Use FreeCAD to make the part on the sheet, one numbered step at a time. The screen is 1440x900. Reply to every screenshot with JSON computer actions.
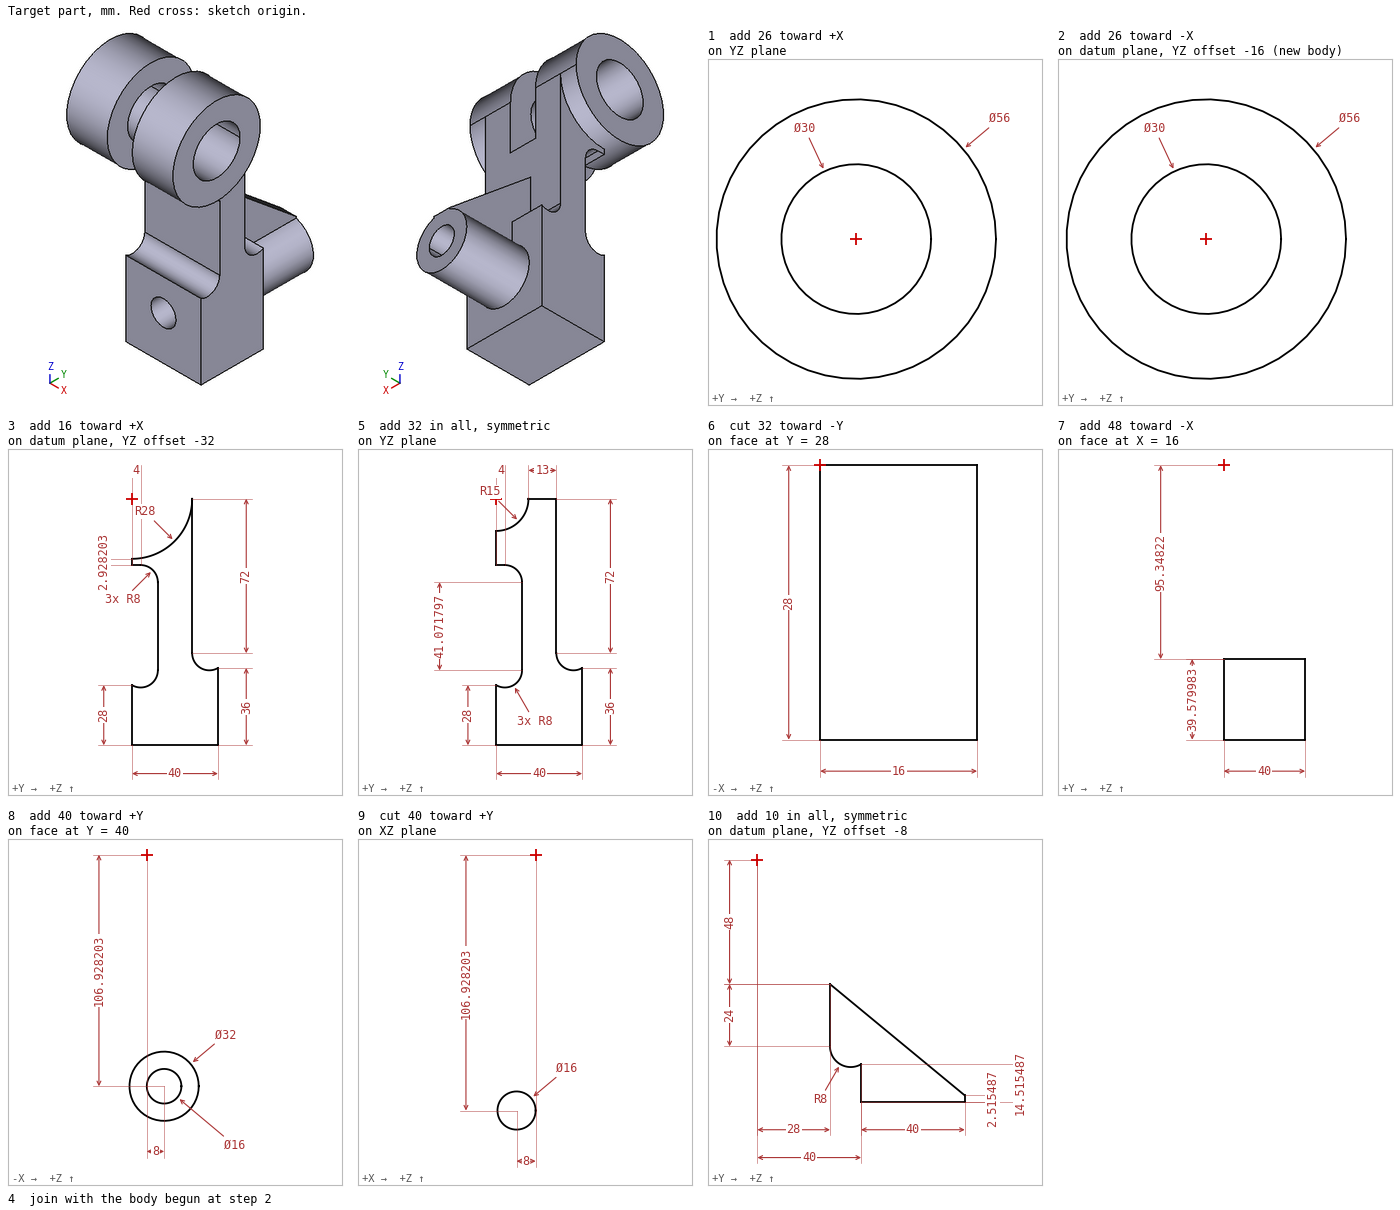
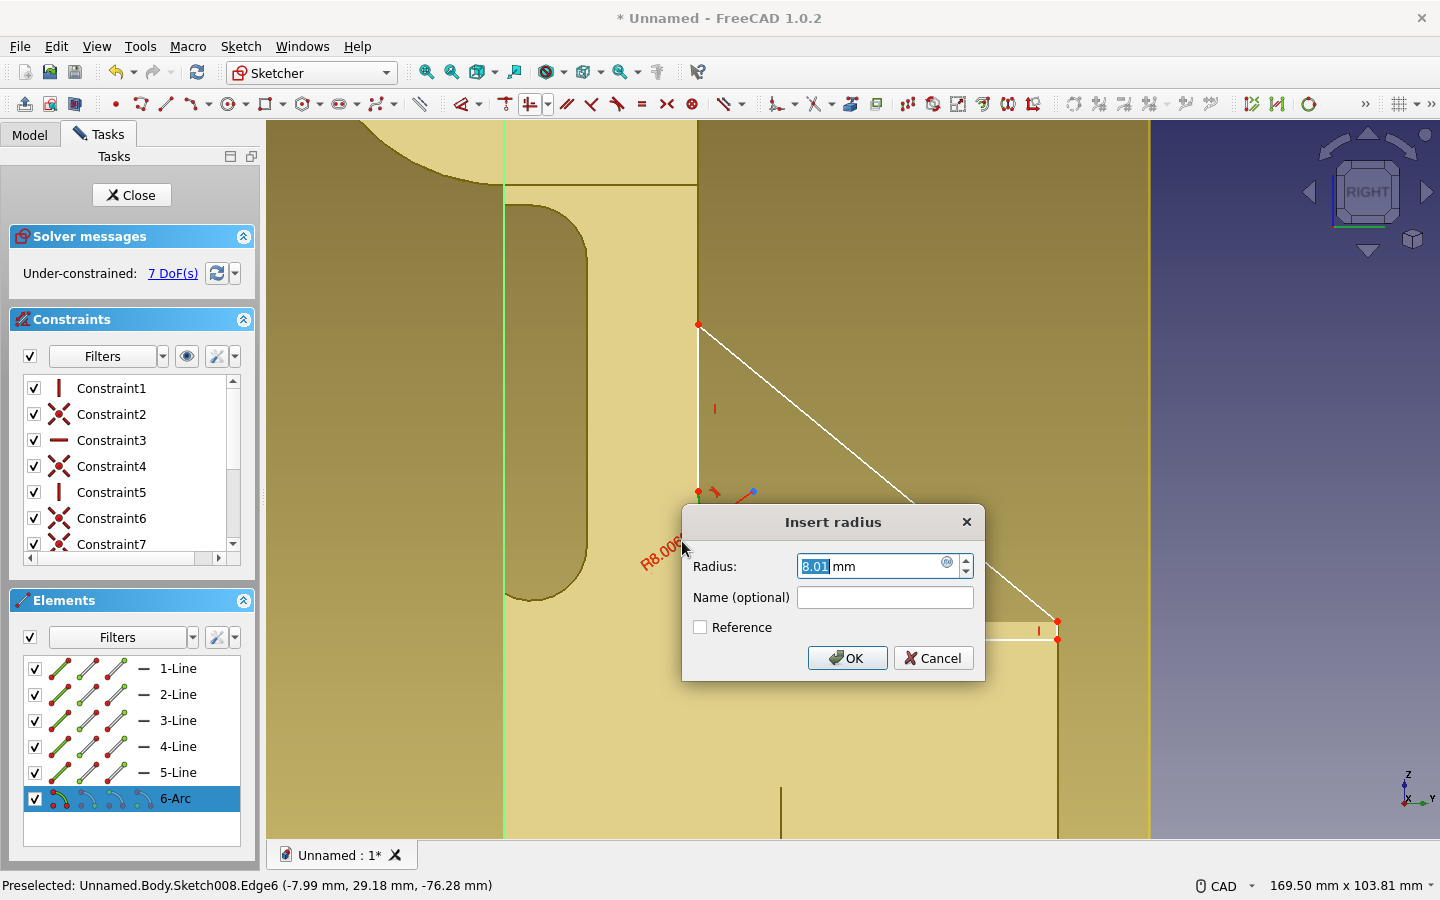
{"action": "type", "text": "8"}
{"action": "key", "text": "Return"}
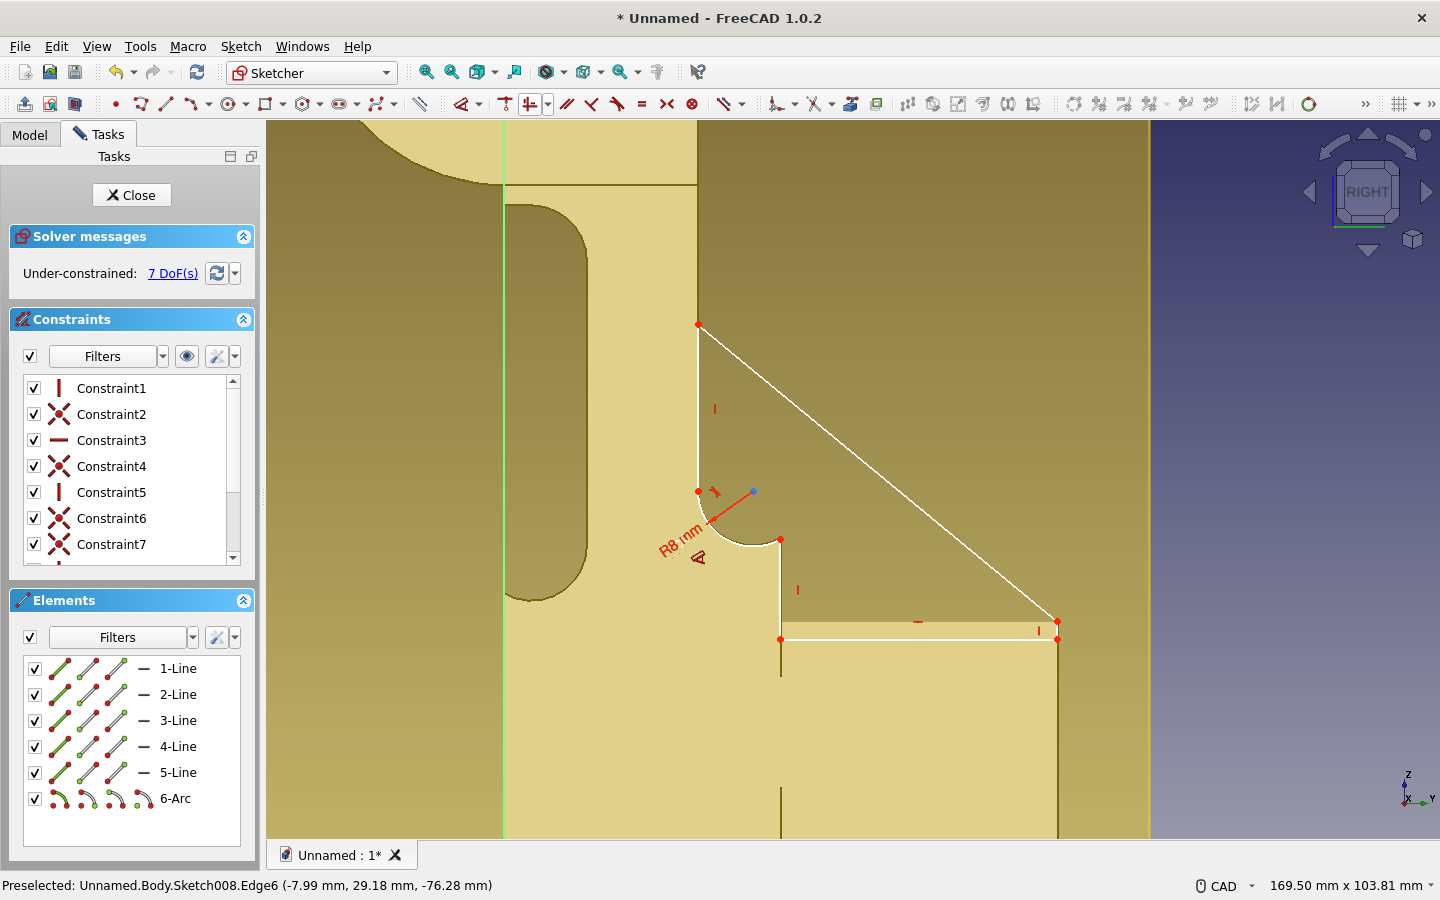
{"action": "left_click", "coordinate": [864, 640]}
{"action": "left_click", "coordinate": [919, 674]}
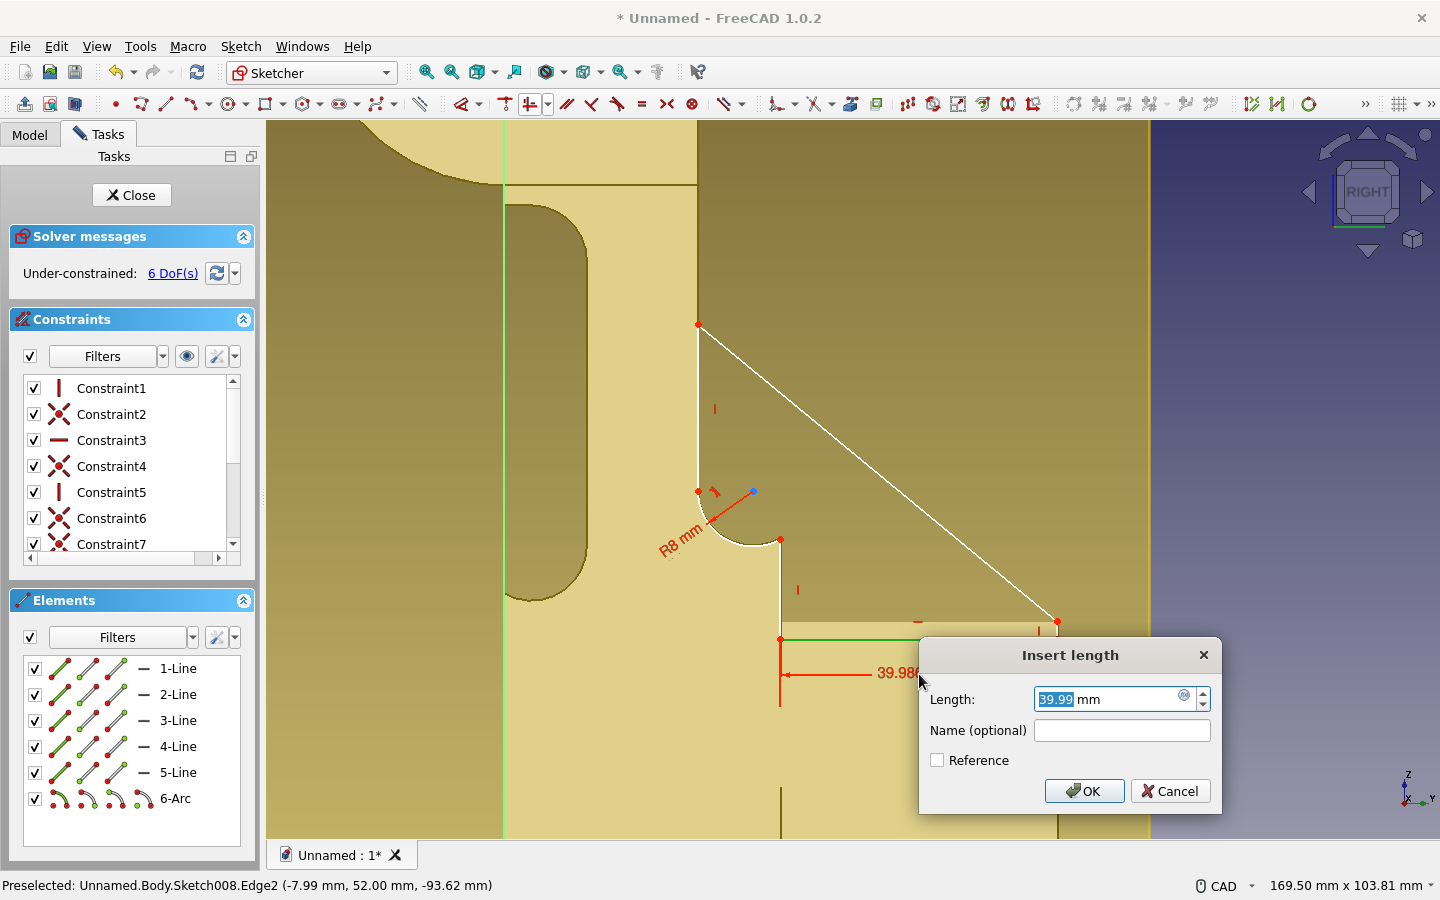
{"action": "type", "text": "40"}
{"action": "key", "text": "Return"}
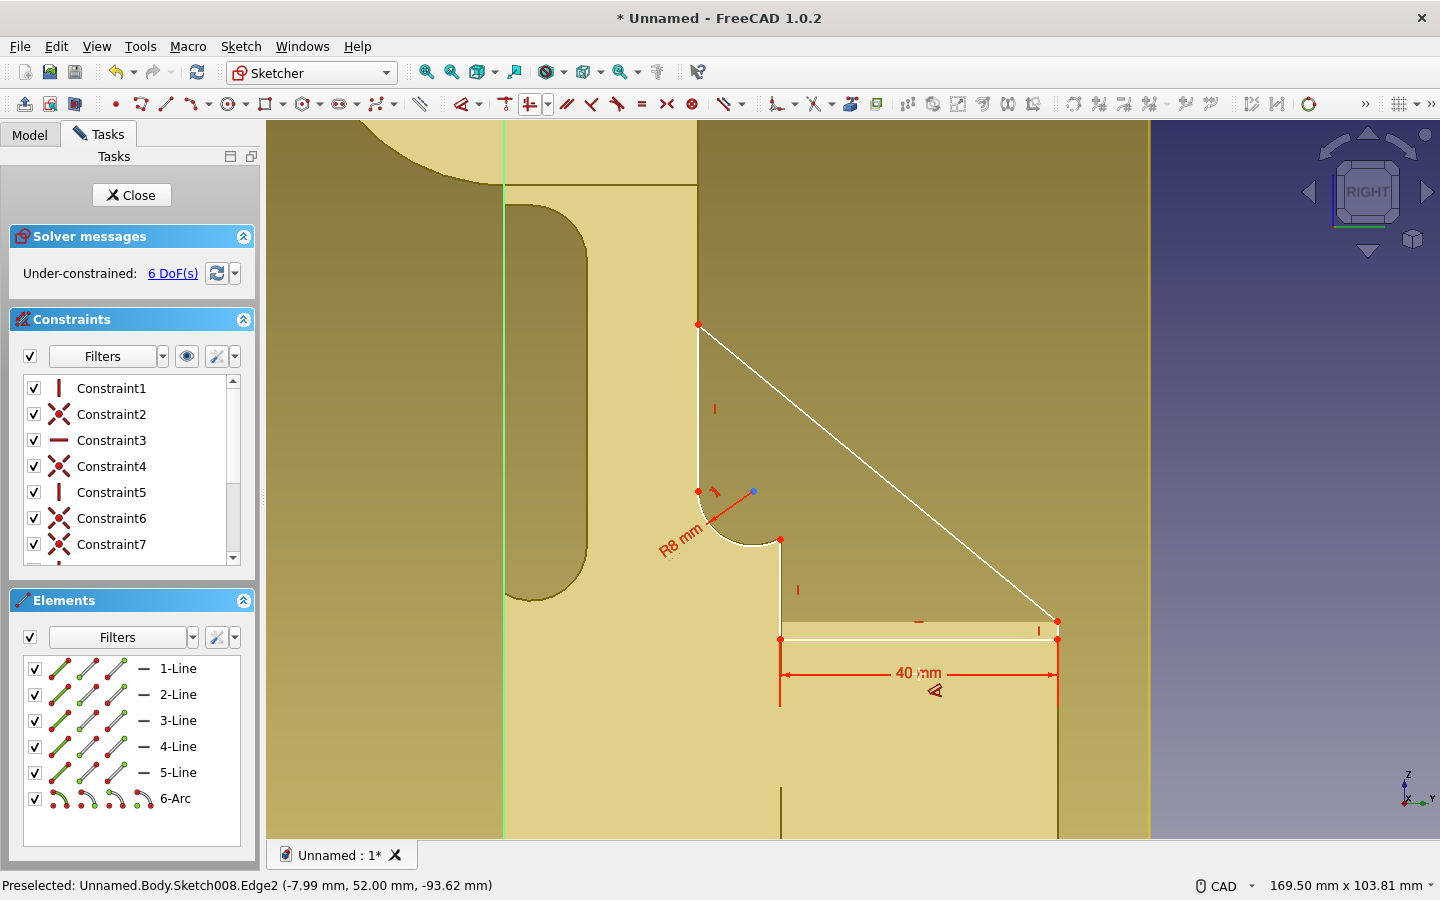
{"action": "left_click", "coordinate": [698, 375]}
{"action": "left_click", "coordinate": [664, 408]}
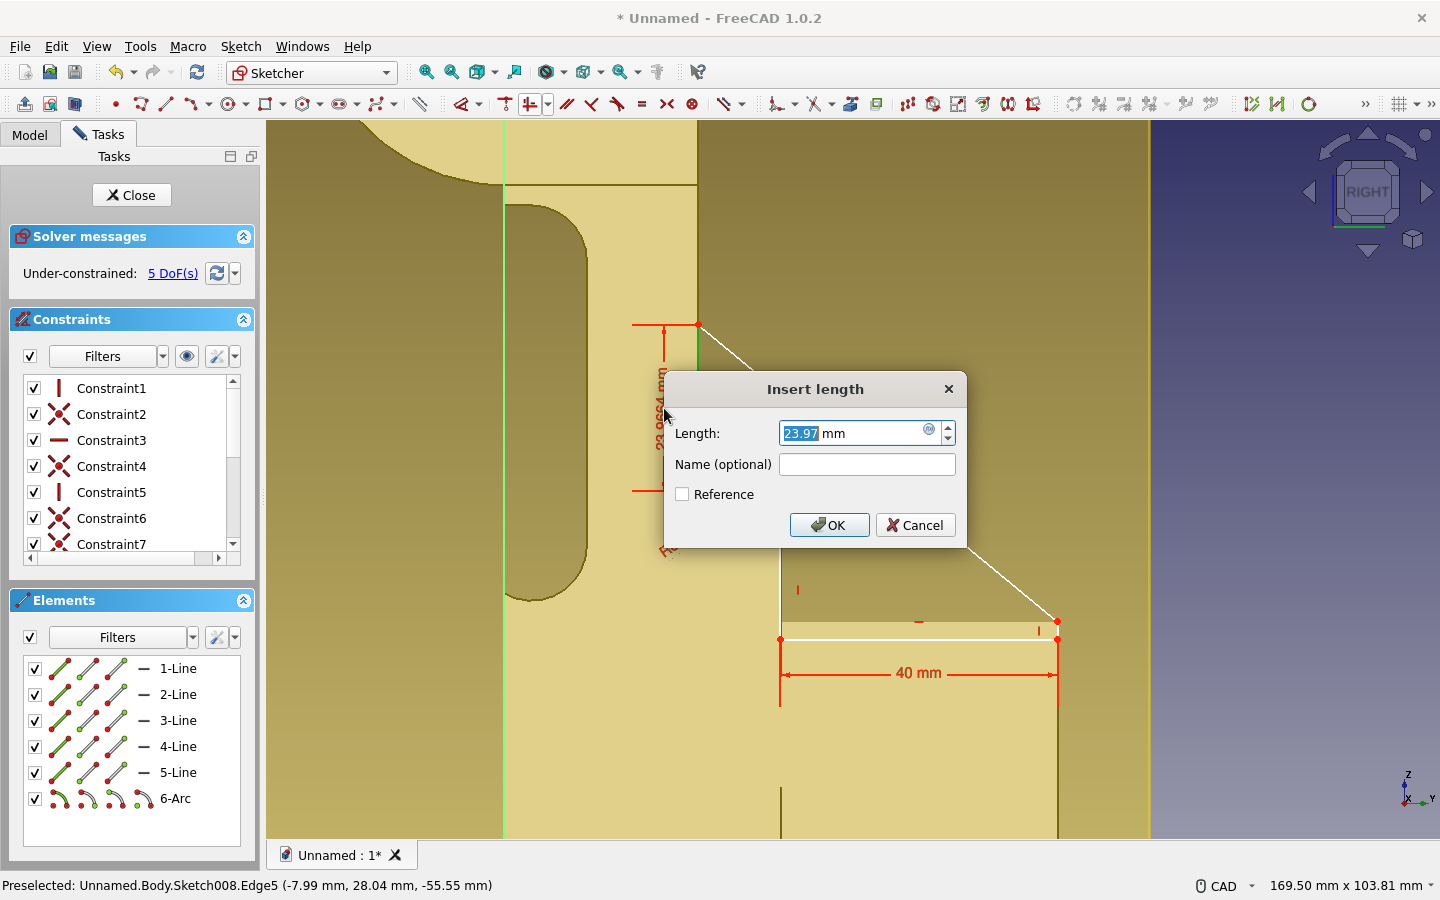
{"action": "type", "text": "24"}
{"action": "key", "text": "Return"}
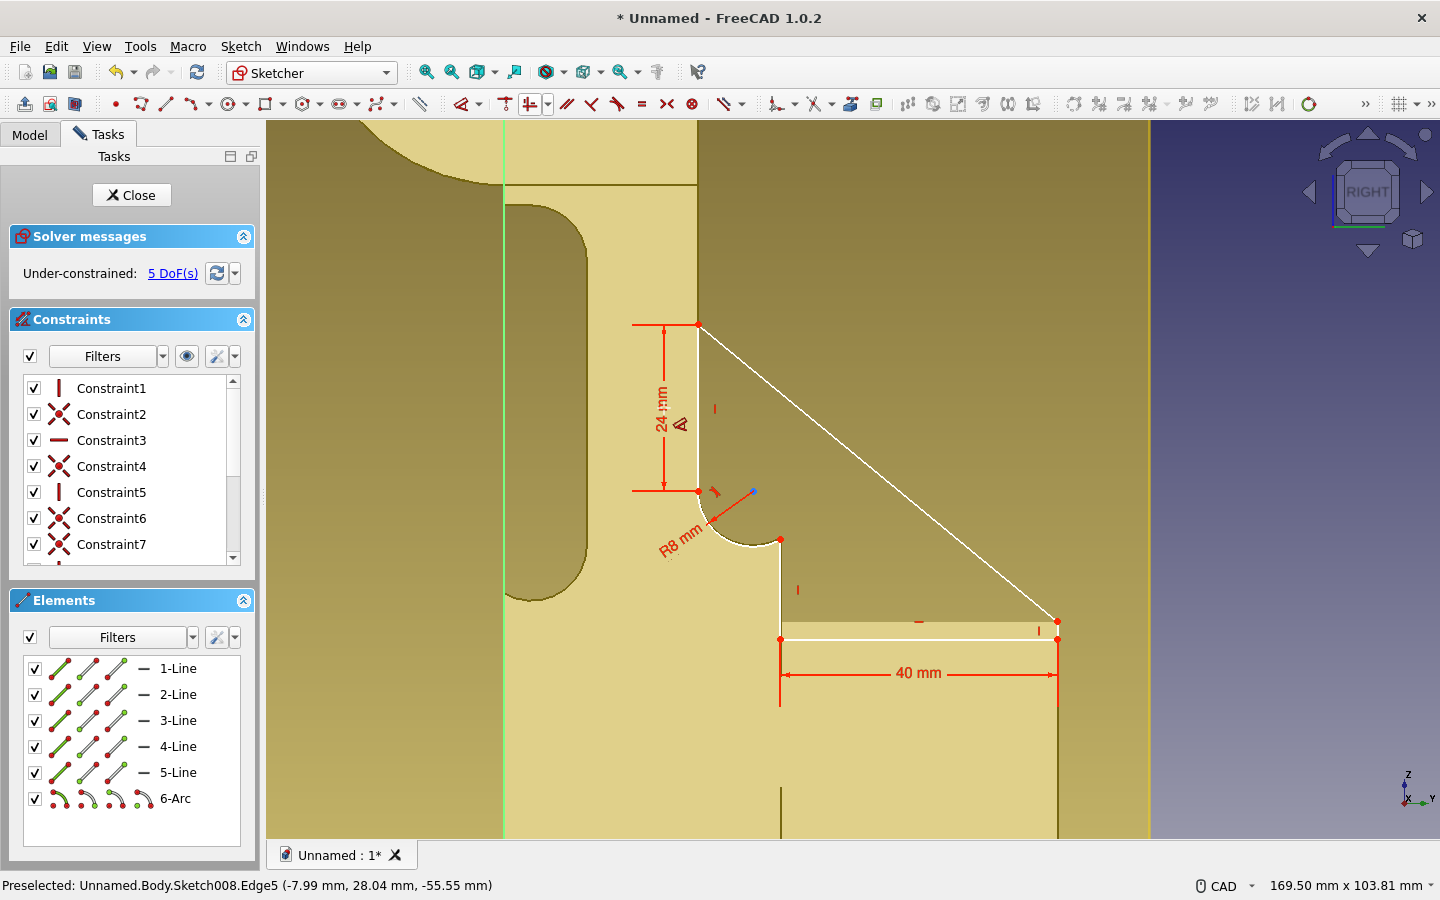
{"action": "left_click", "coordinate": [780, 540]}
{"action": "left_click", "coordinate": [642, 574]}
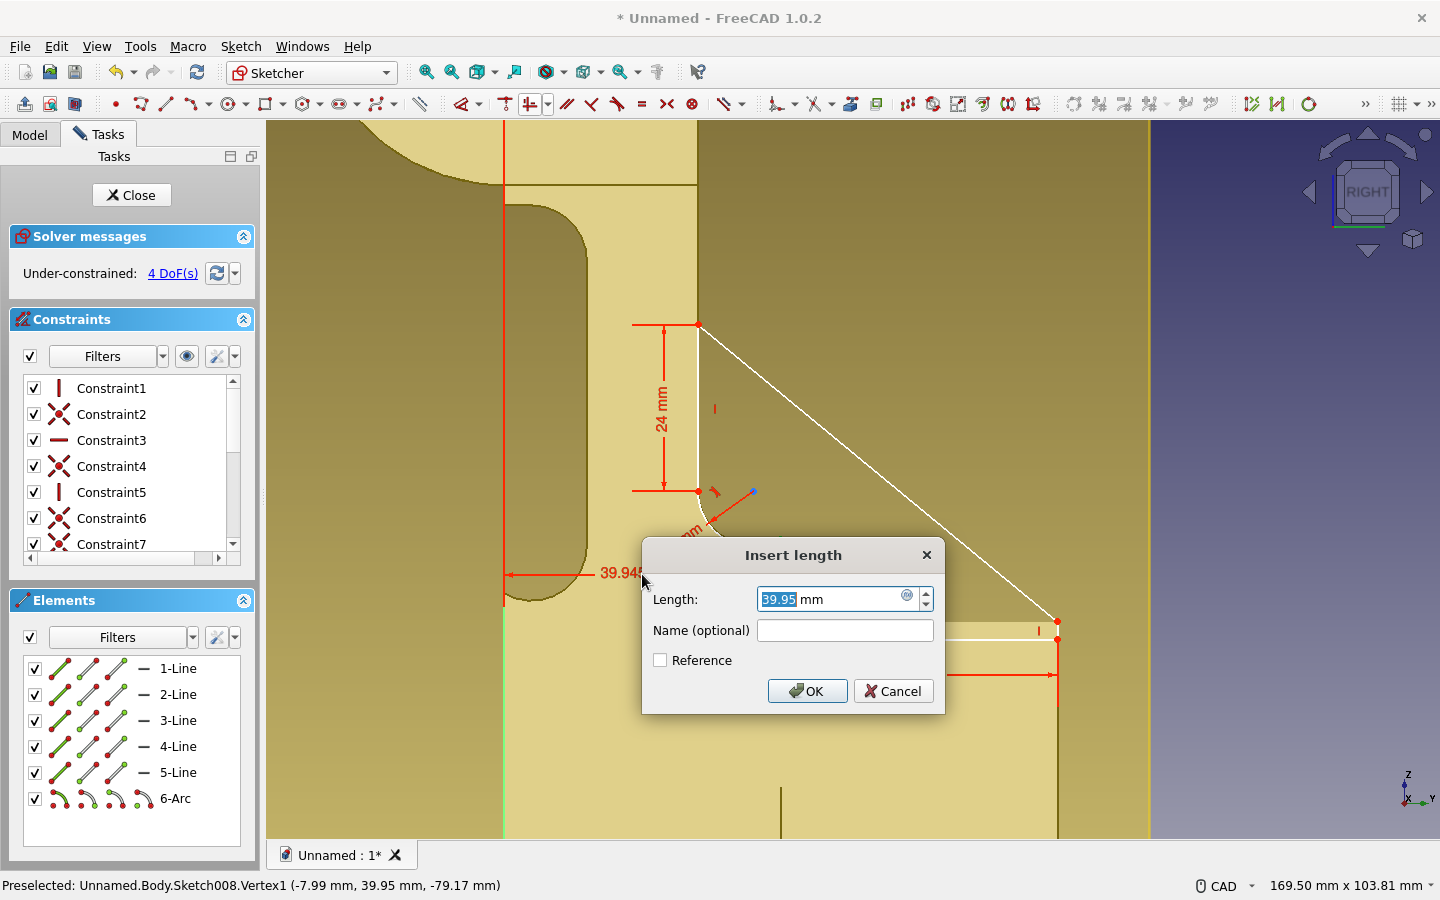
{"action": "type", "text": "40"}
{"action": "key", "text": "Return"}